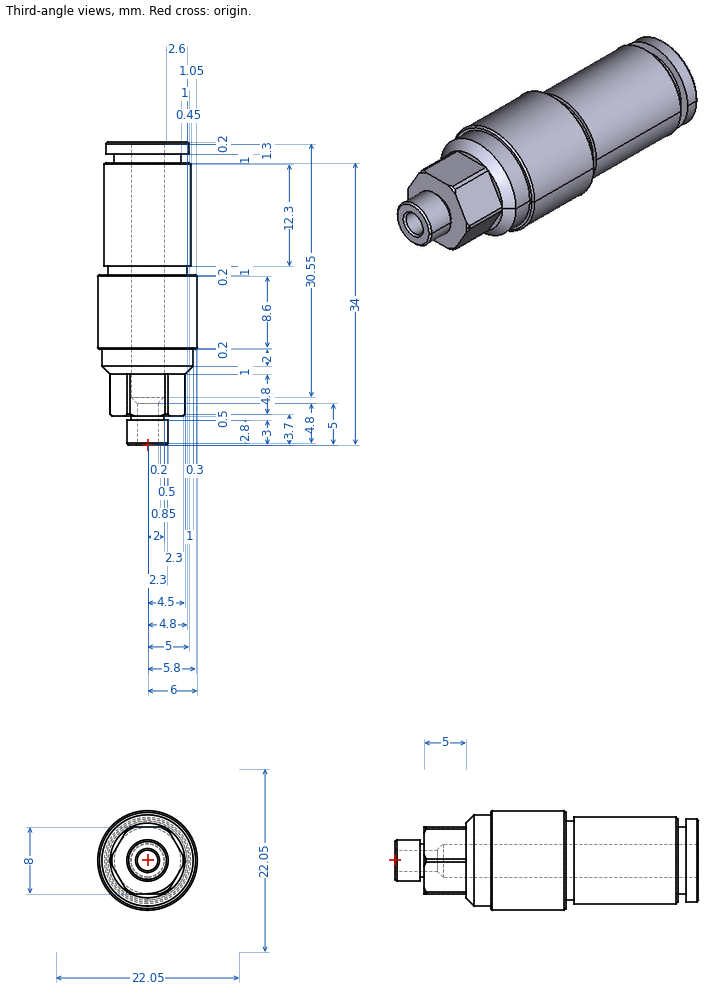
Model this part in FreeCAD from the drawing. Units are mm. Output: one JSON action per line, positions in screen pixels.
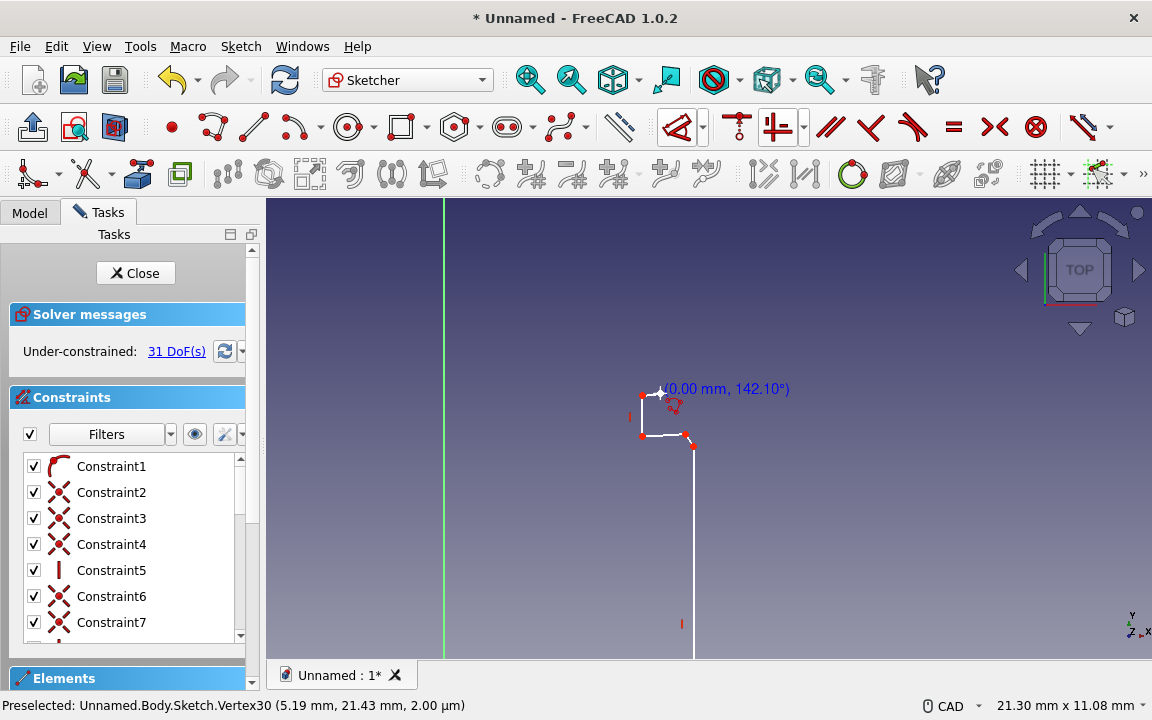
{"action": "scroll", "coordinate": [659, 404], "scroll_direction": "down", "scroll_amount": 8}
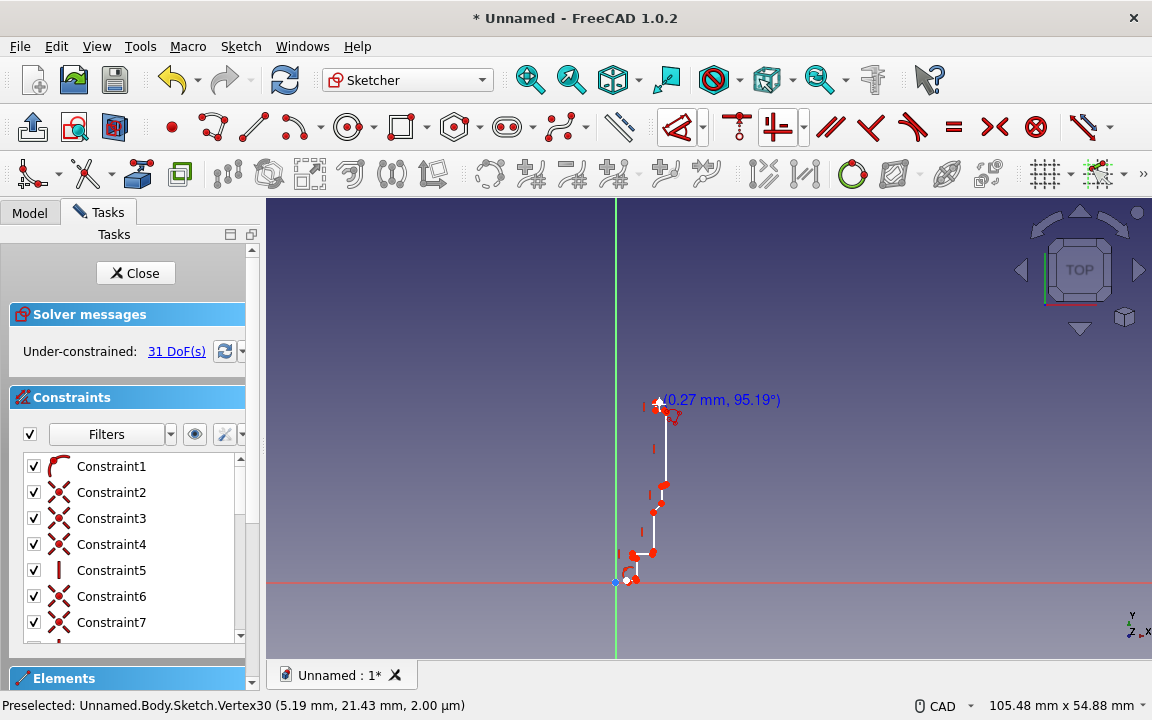
{"action": "left_click", "coordinate": [660, 299]}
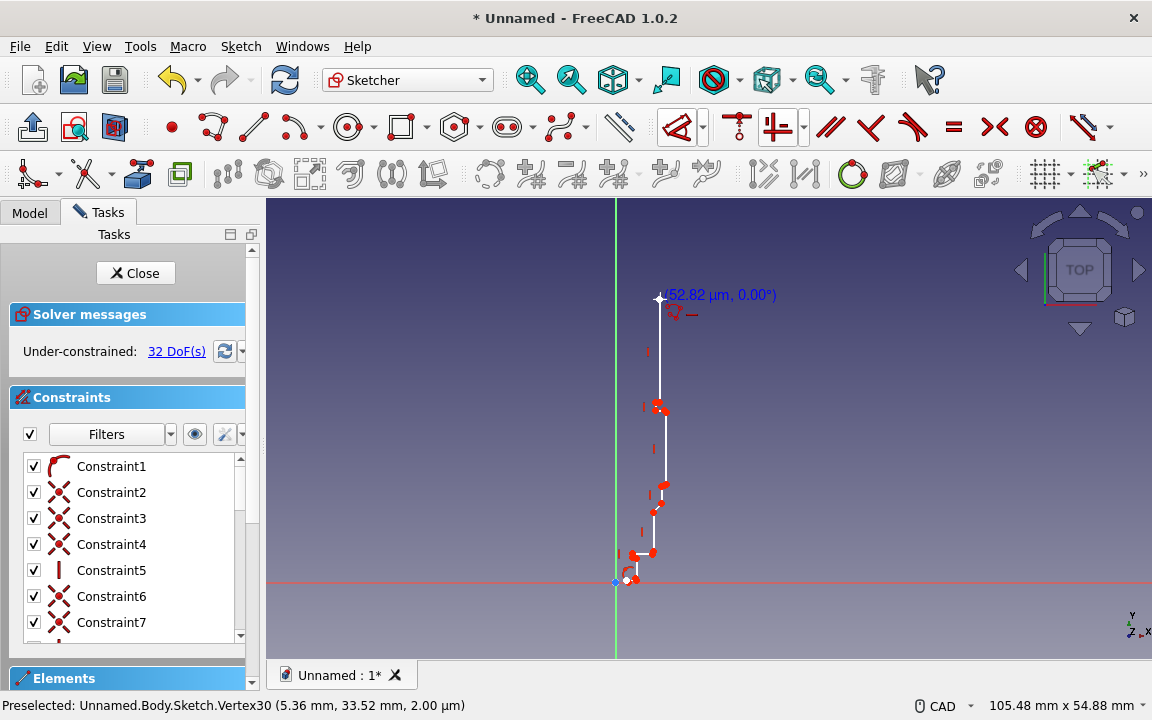
{"action": "scroll", "coordinate": [658, 297], "scroll_direction": "up", "scroll_amount": 10}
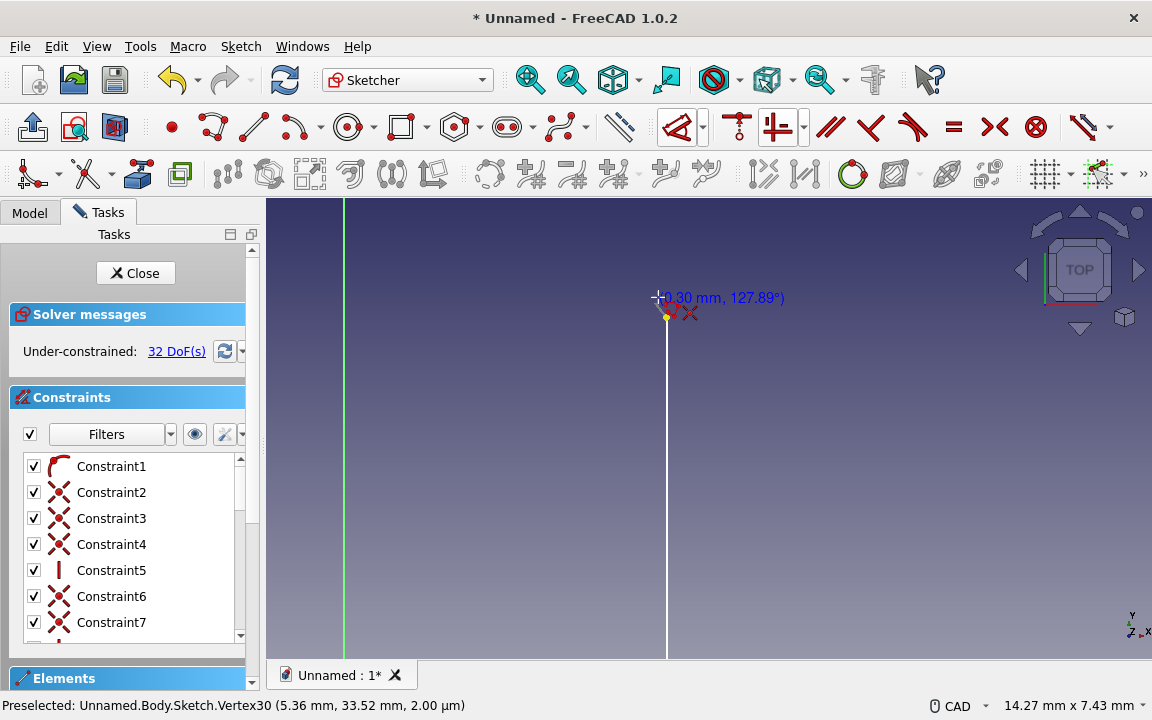
{"action": "left_click", "coordinate": [655, 295]}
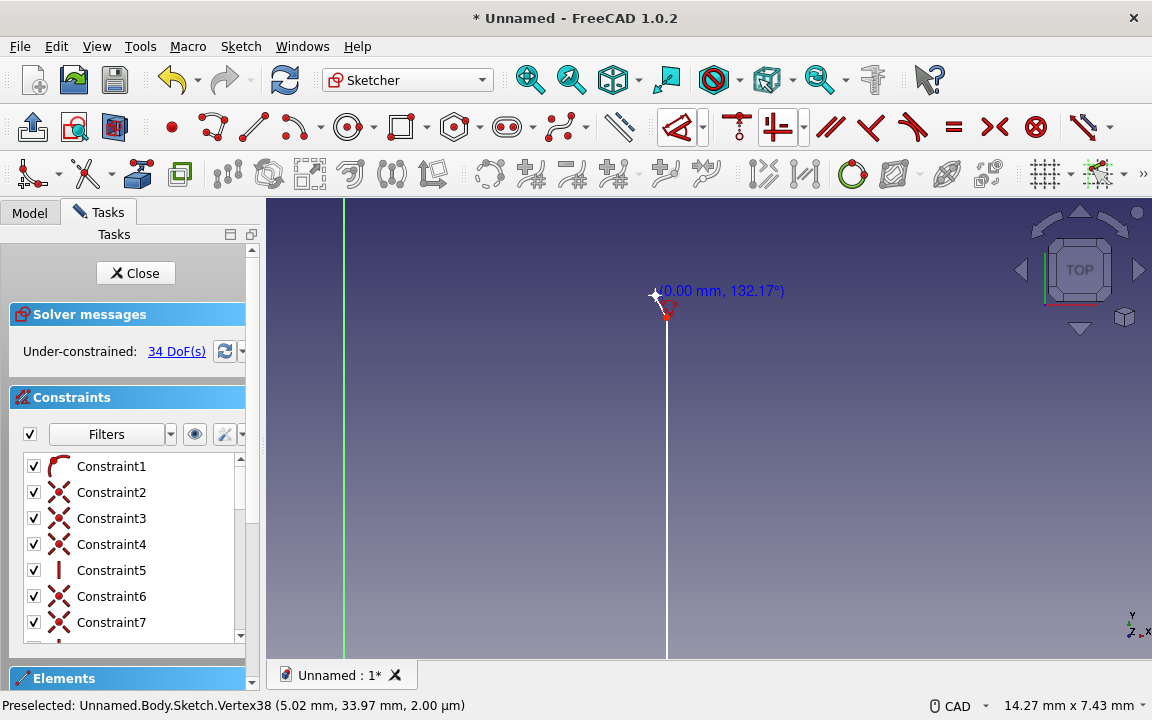
{"action": "scroll", "coordinate": [658, 296], "scroll_direction": "down", "scroll_amount": 10}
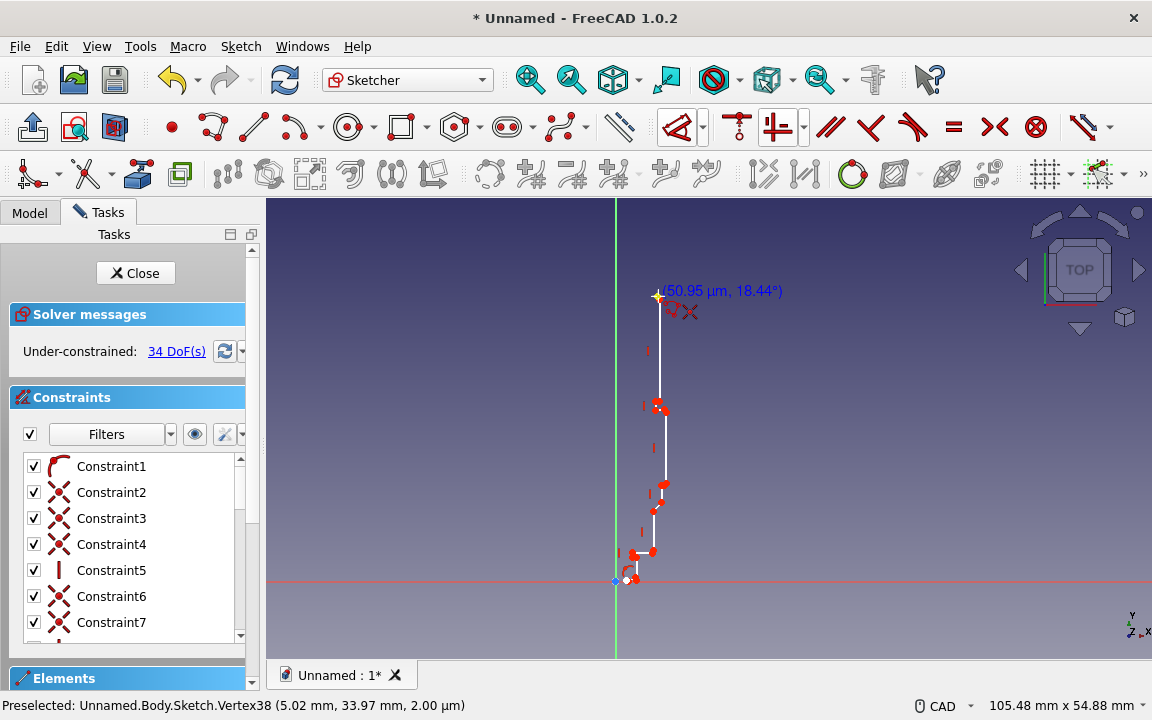
{"action": "scroll", "coordinate": [650, 296], "scroll_direction": "up", "scroll_amount": 4}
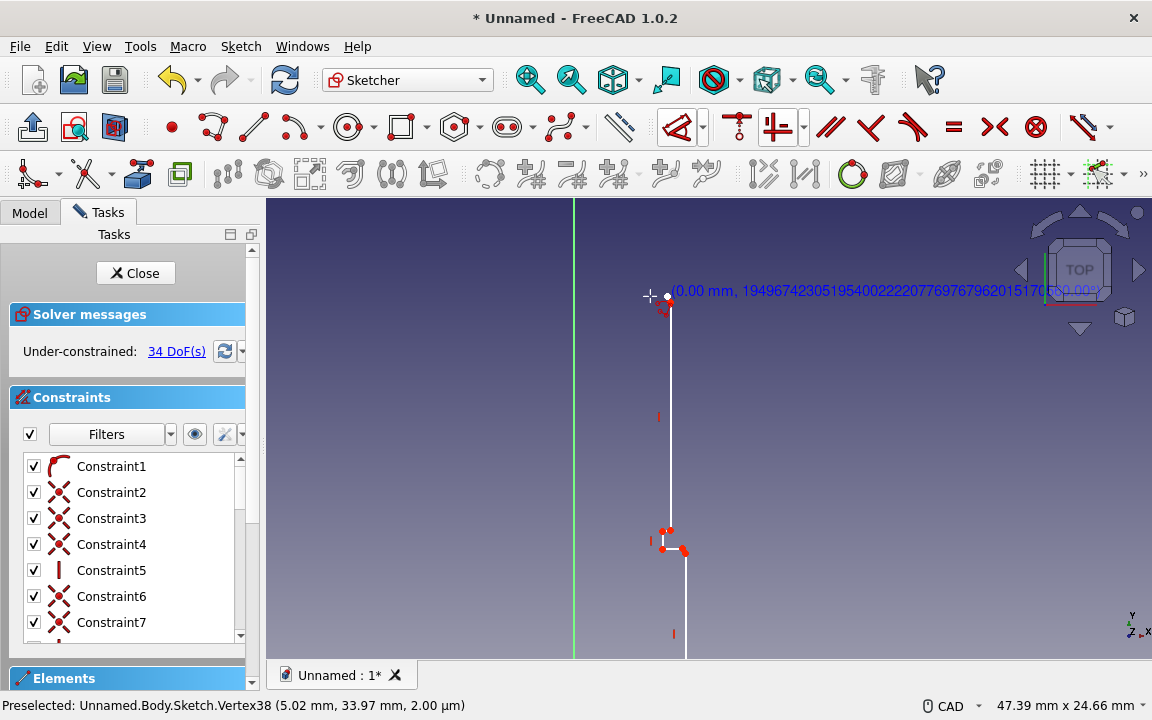
{"action": "left_click", "coordinate": [648, 296]}
{"action": "left_click", "coordinate": [648, 277]}
{"action": "left_click", "coordinate": [667, 277]}
{"action": "left_click", "coordinate": [667, 253]}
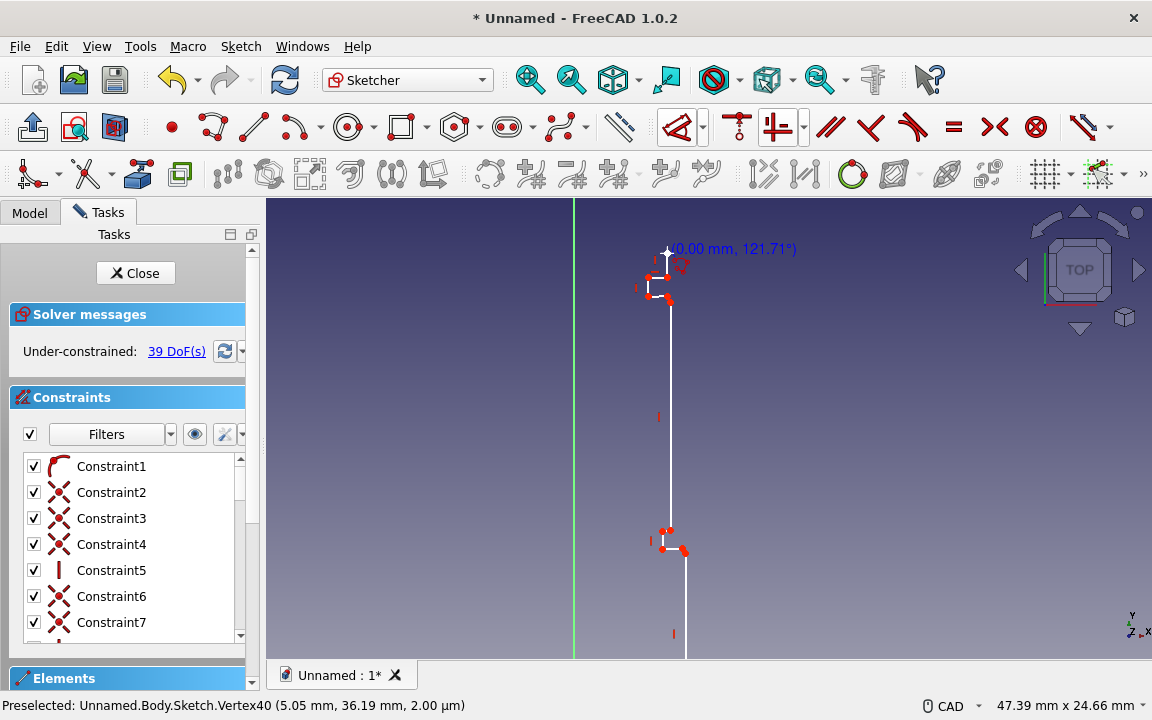
{"action": "scroll", "coordinate": [663, 249], "scroll_direction": "up", "scroll_amount": 6}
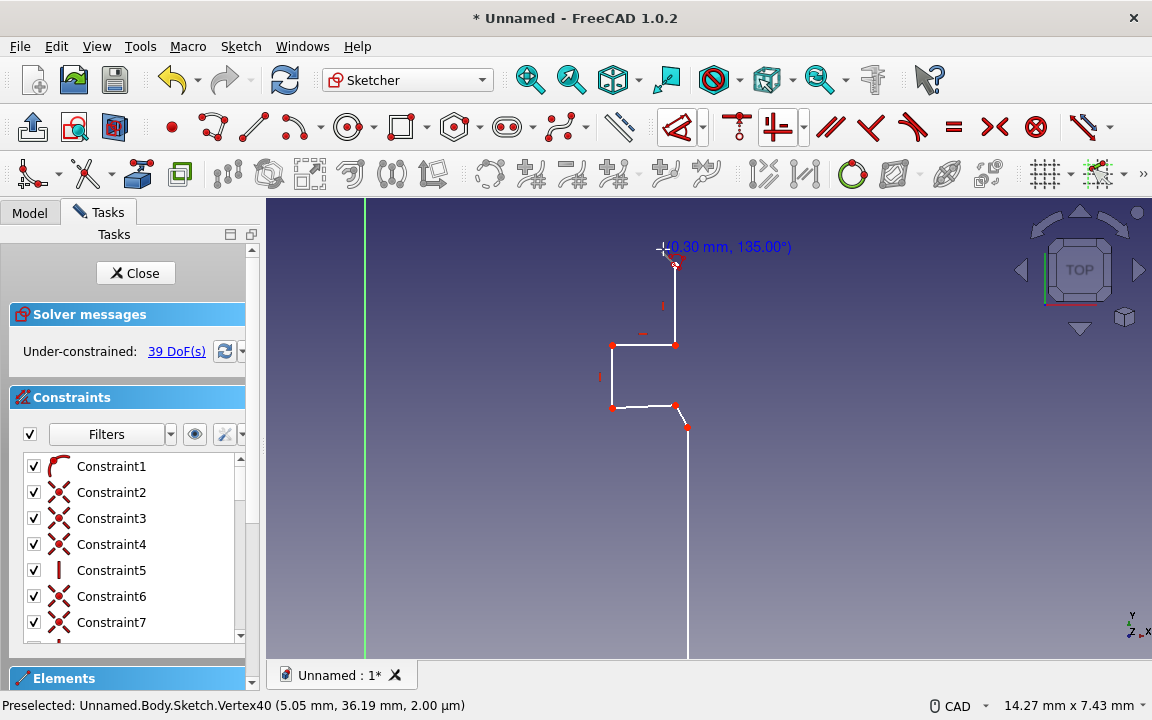
{"action": "left_click", "coordinate": [663, 249]}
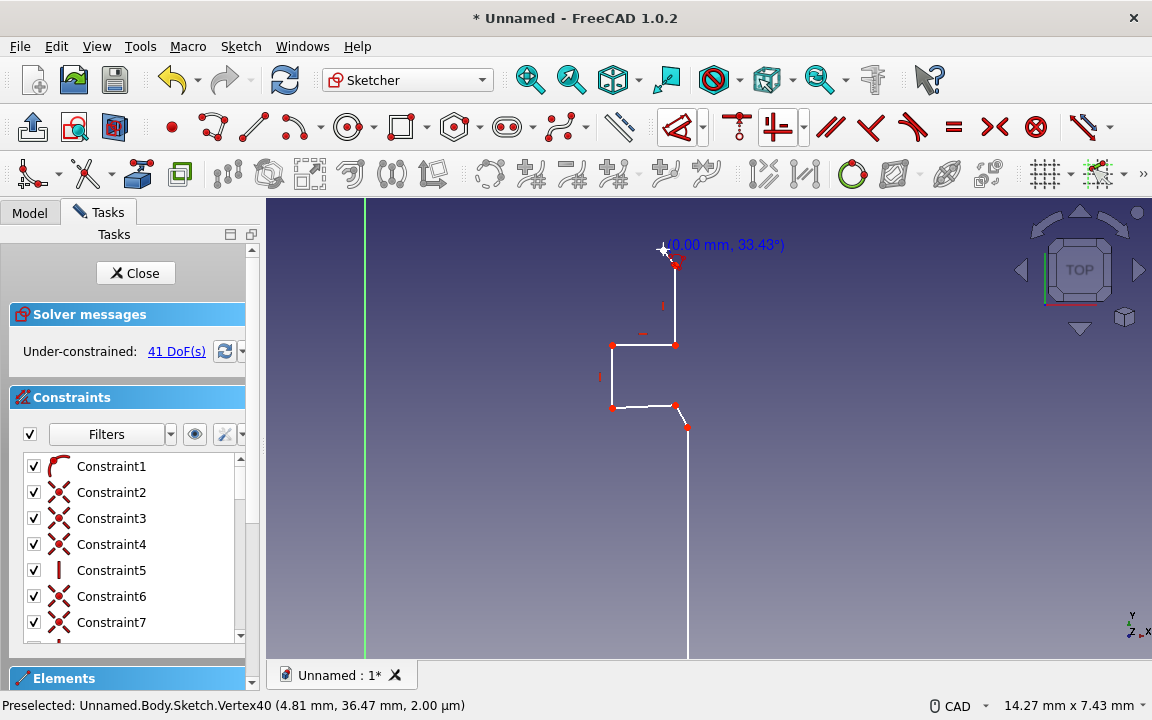
{"action": "scroll", "coordinate": [654, 279], "scroll_direction": "down", "scroll_amount": 10}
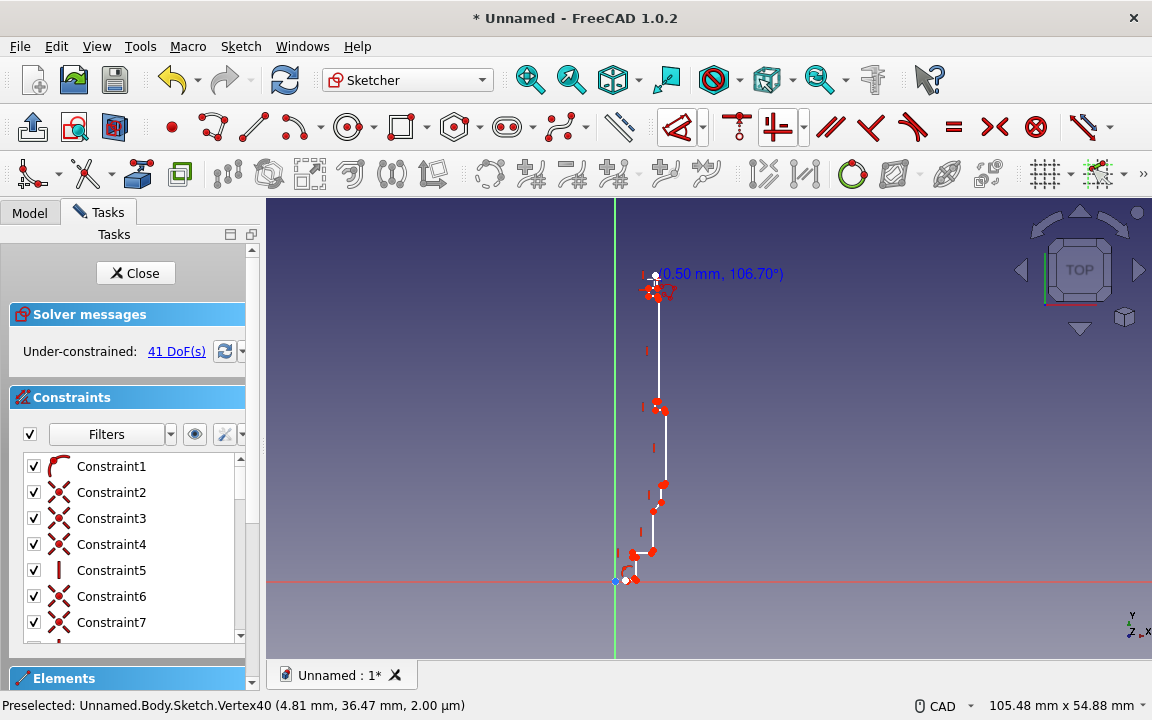
{"action": "left_click", "coordinate": [634, 275]}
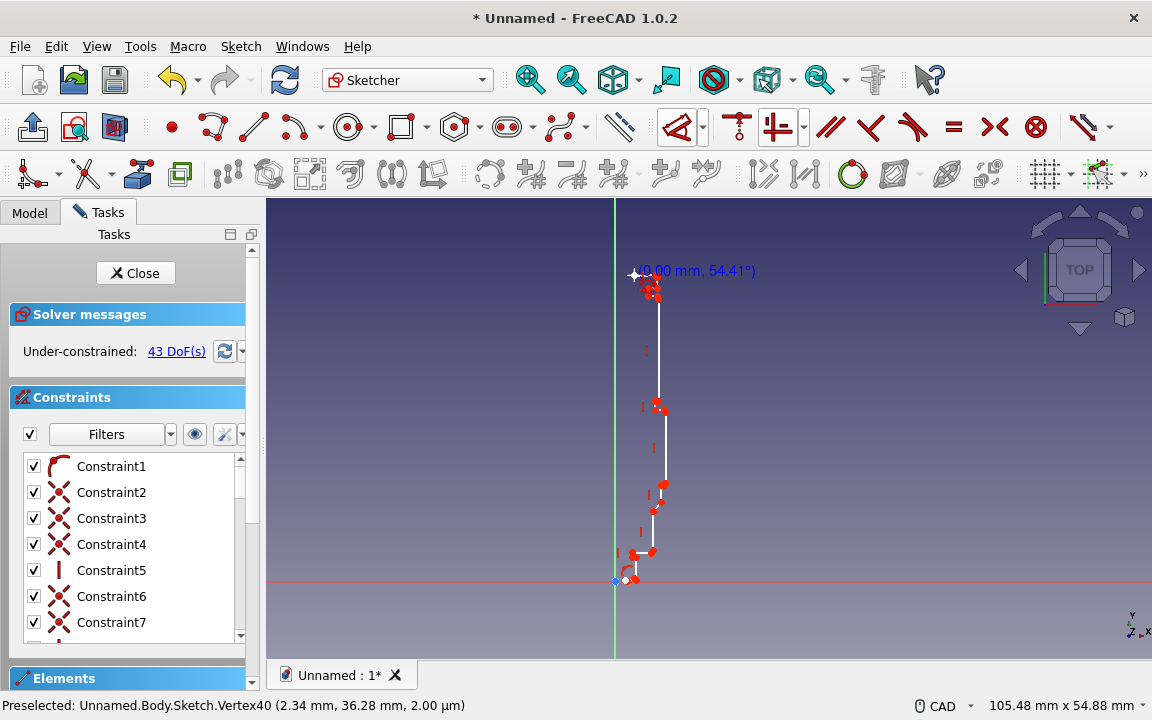
{"action": "scroll", "coordinate": [632, 277], "scroll_direction": "up", "scroll_amount": 10}